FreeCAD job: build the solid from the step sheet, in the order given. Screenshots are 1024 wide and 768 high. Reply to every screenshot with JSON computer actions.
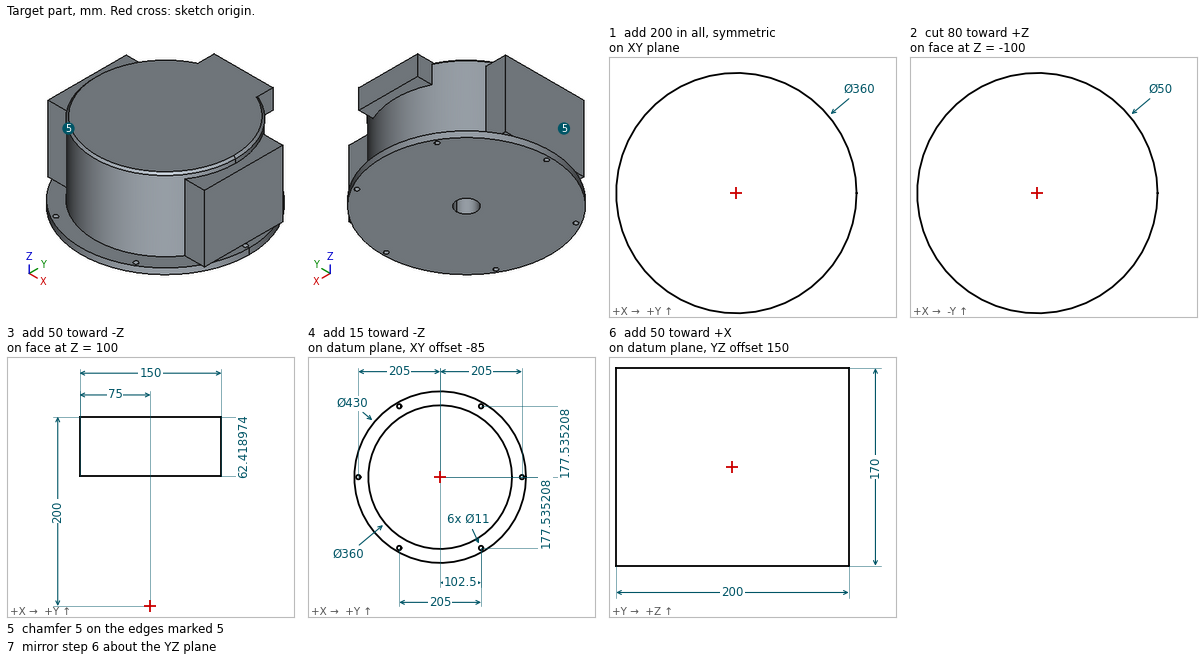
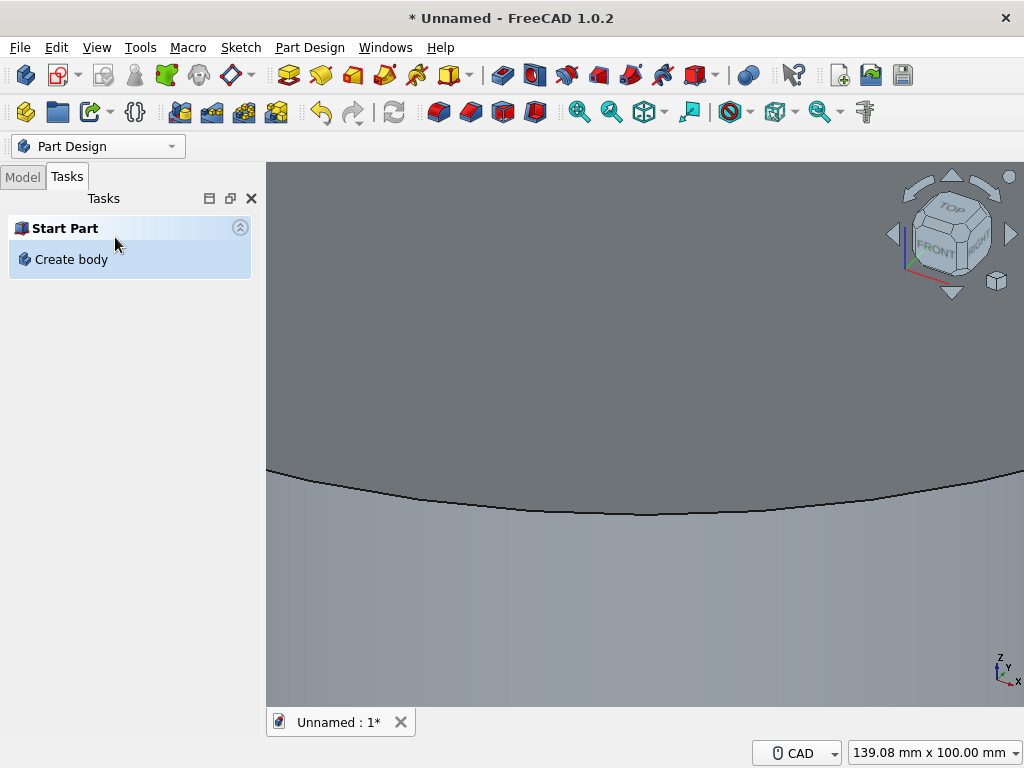
{"action": "left_click", "coordinate": [580, 112]}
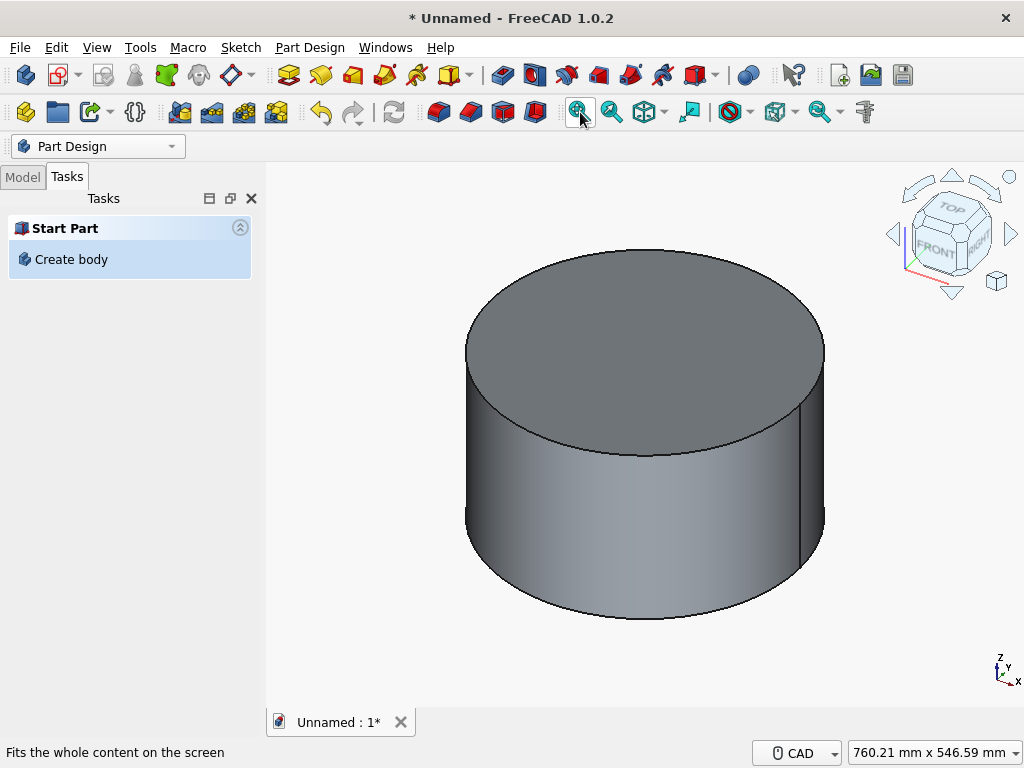
{"action": "key", "text": "5"}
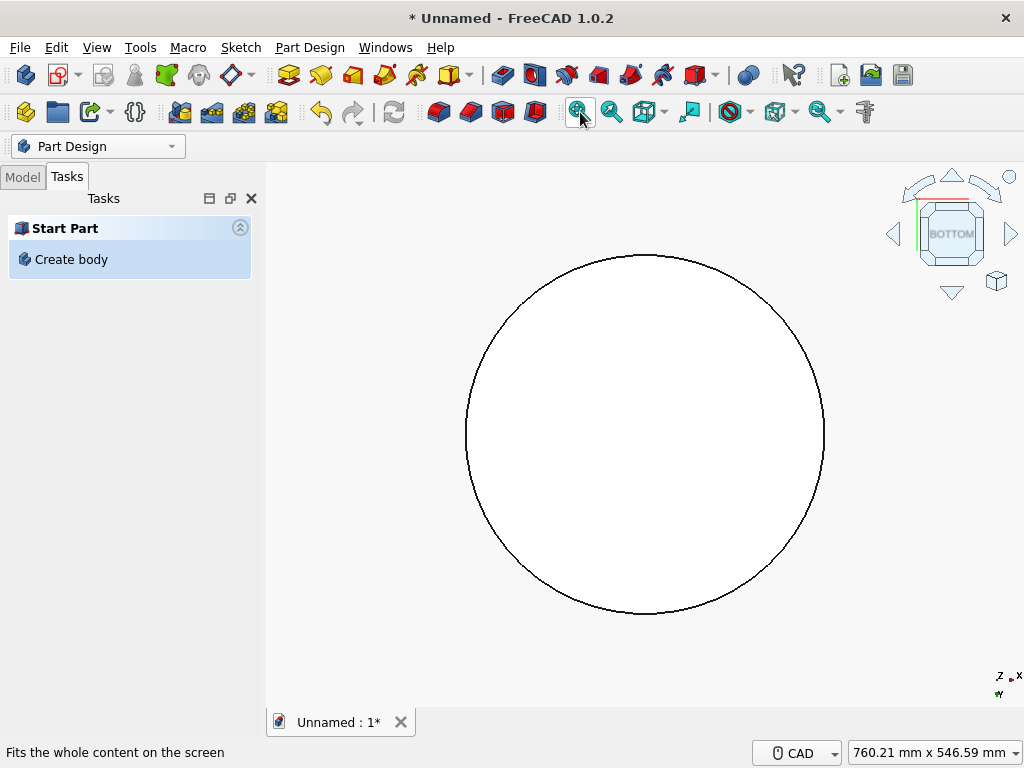
{"action": "left_click", "coordinate": [645, 433]}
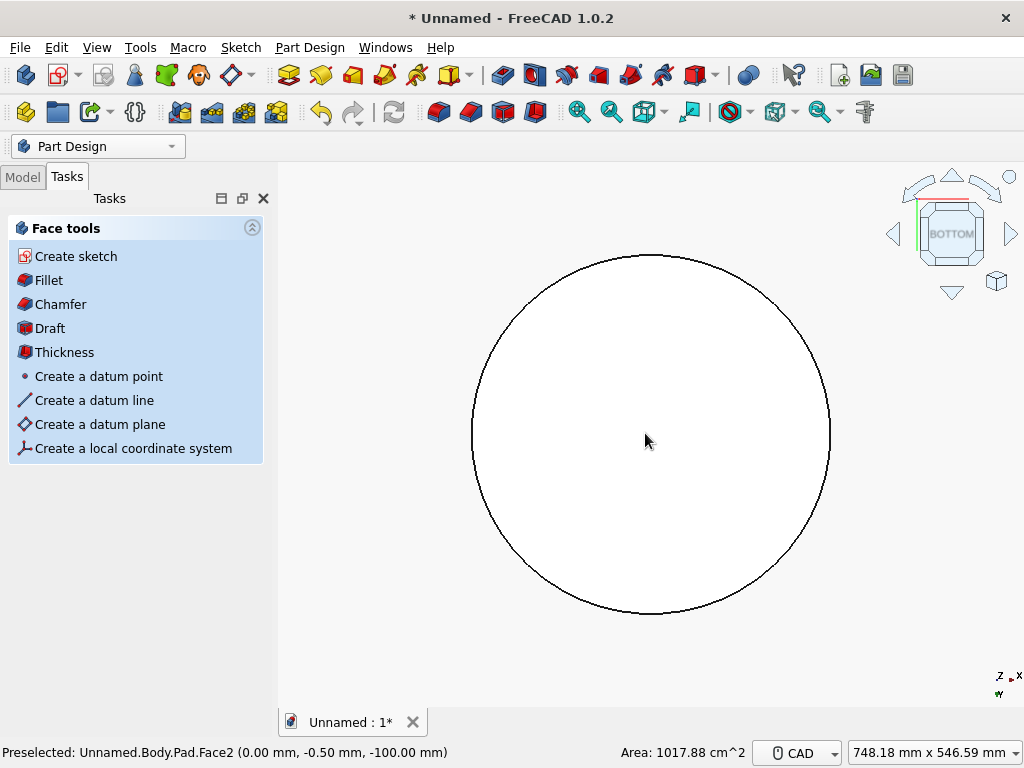
{"action": "left_click", "coordinate": [58, 76]}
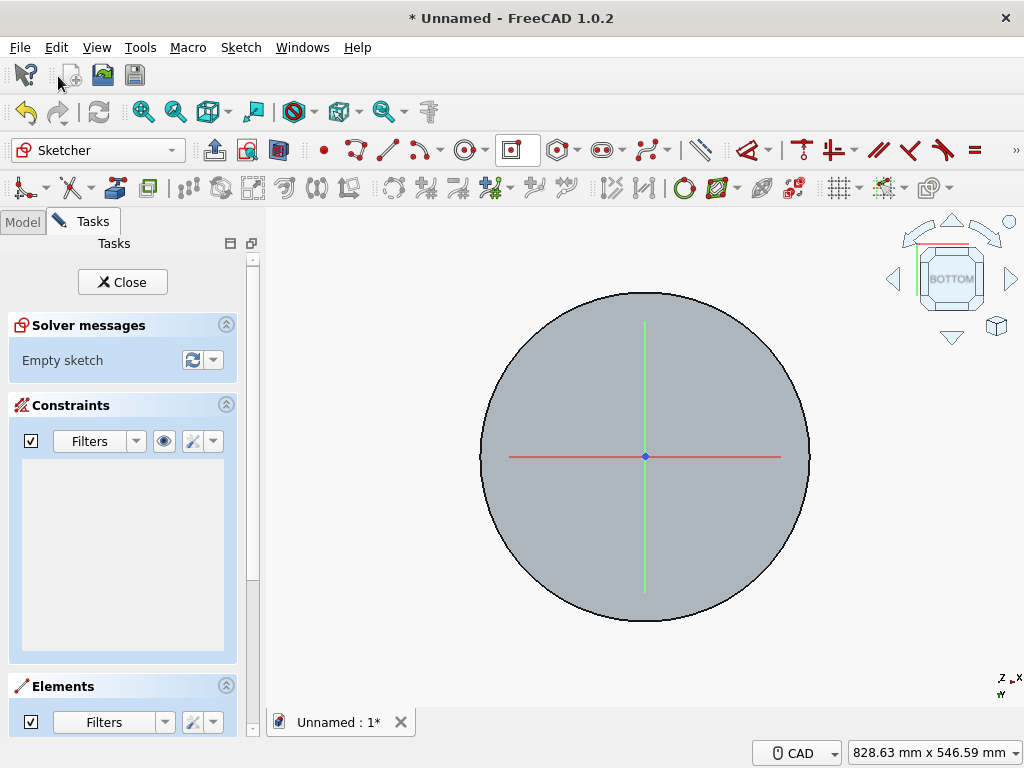
{"action": "scroll", "coordinate": [656, 457], "scroll_direction": "up", "scroll_amount": 10}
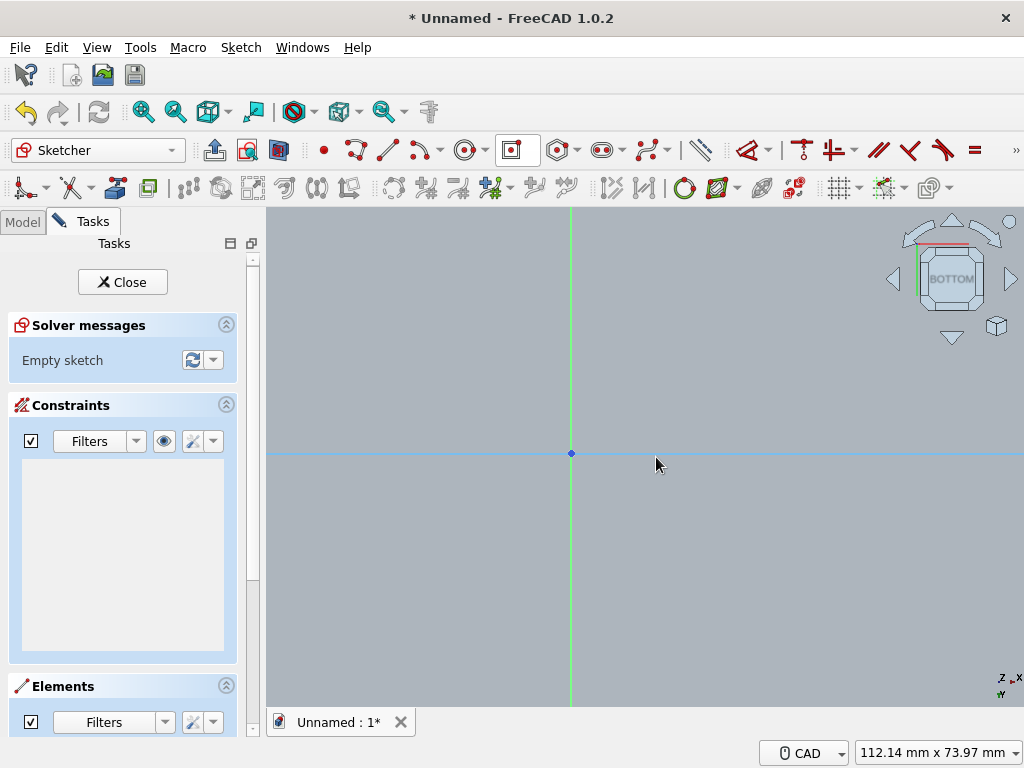
{"action": "key", "text": "g c"}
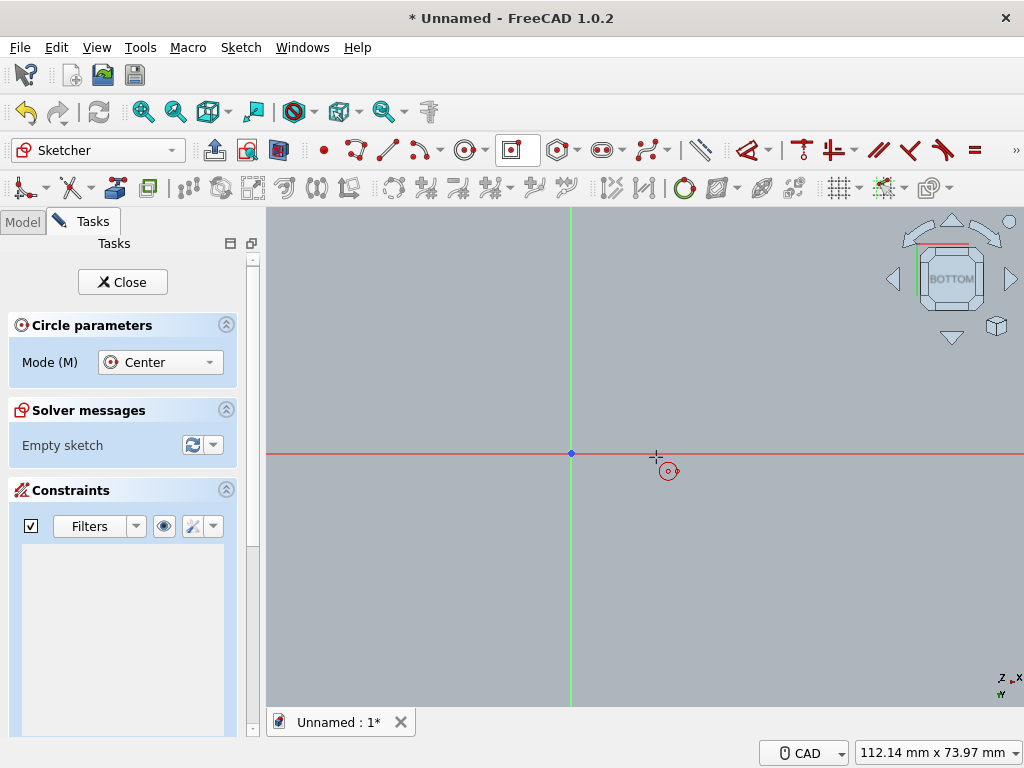
{"action": "left_click", "coordinate": [571, 454]}
{"action": "mouse_move", "coordinate": [691, 334]}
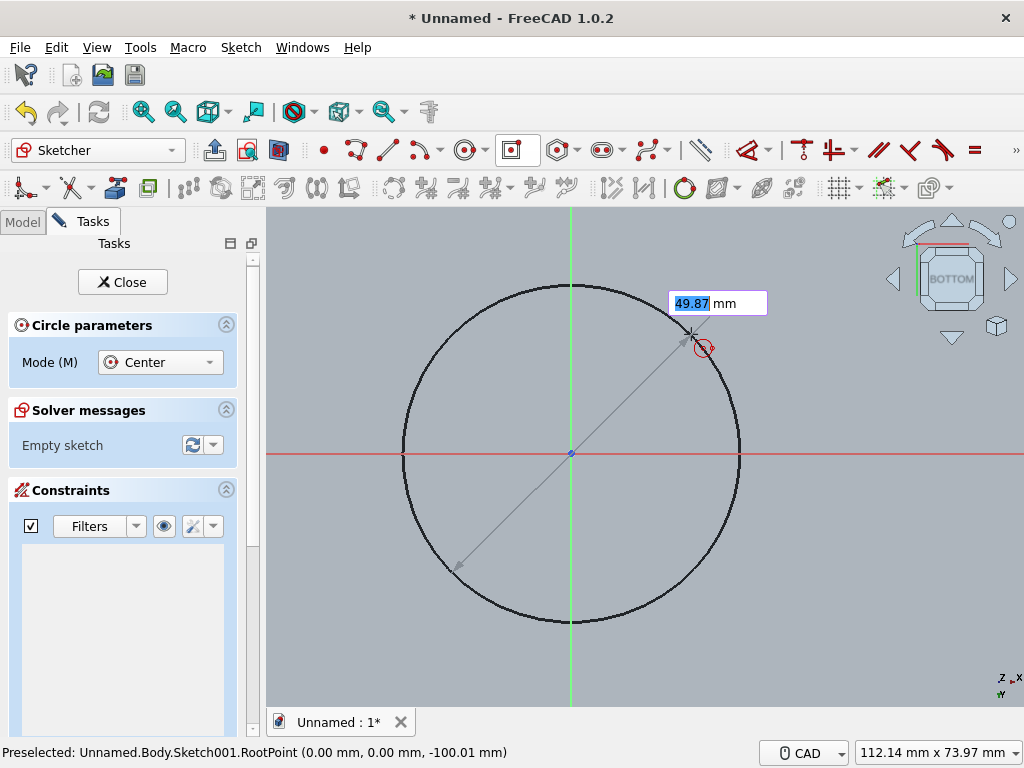
{"action": "type", "text": "50"}
{"action": "key", "text": "Return"}
{"action": "key", "text": "Escape"}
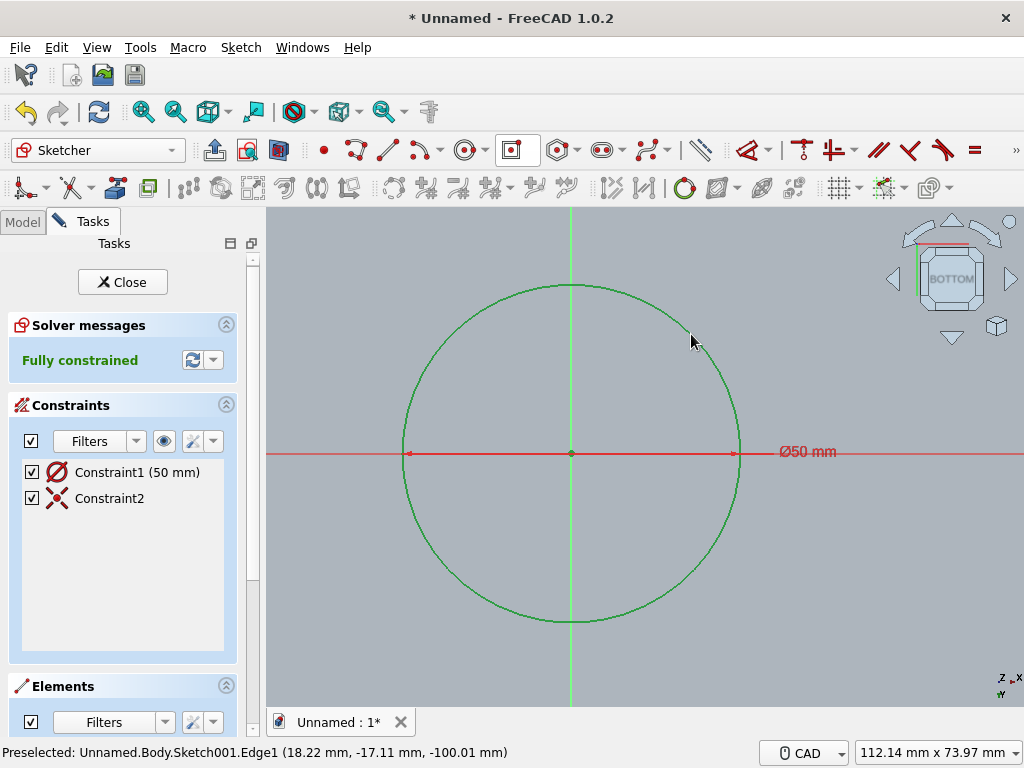
{"action": "left_click", "coordinate": [123, 282]}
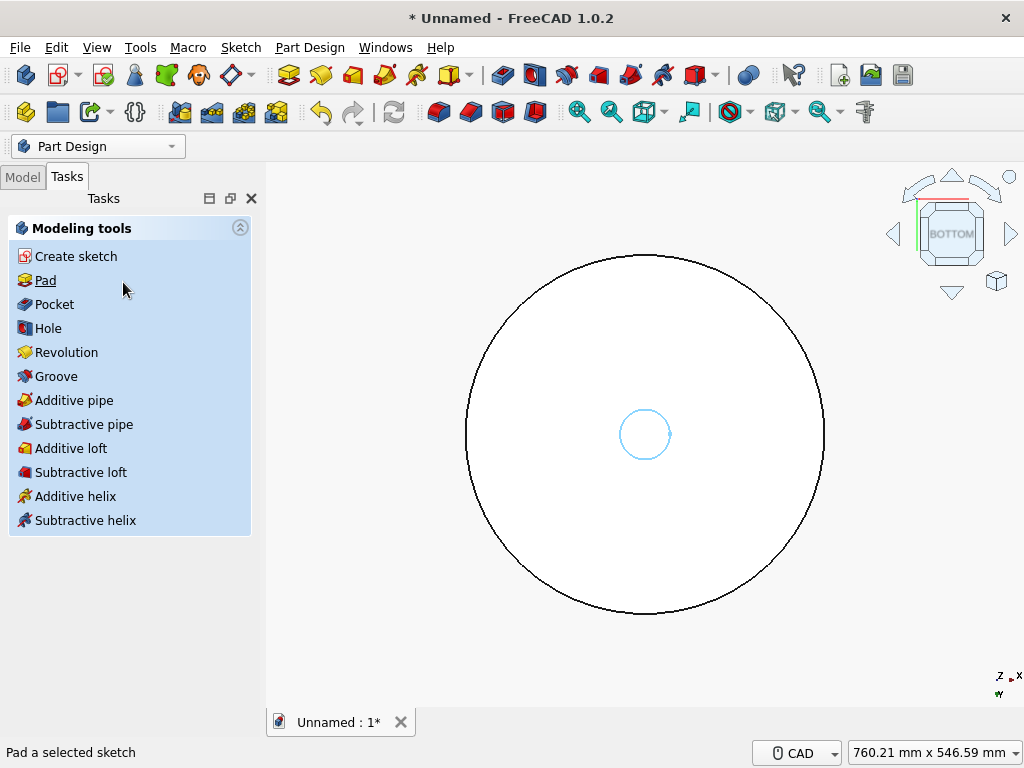
{"action": "left_click", "coordinate": [504, 76]}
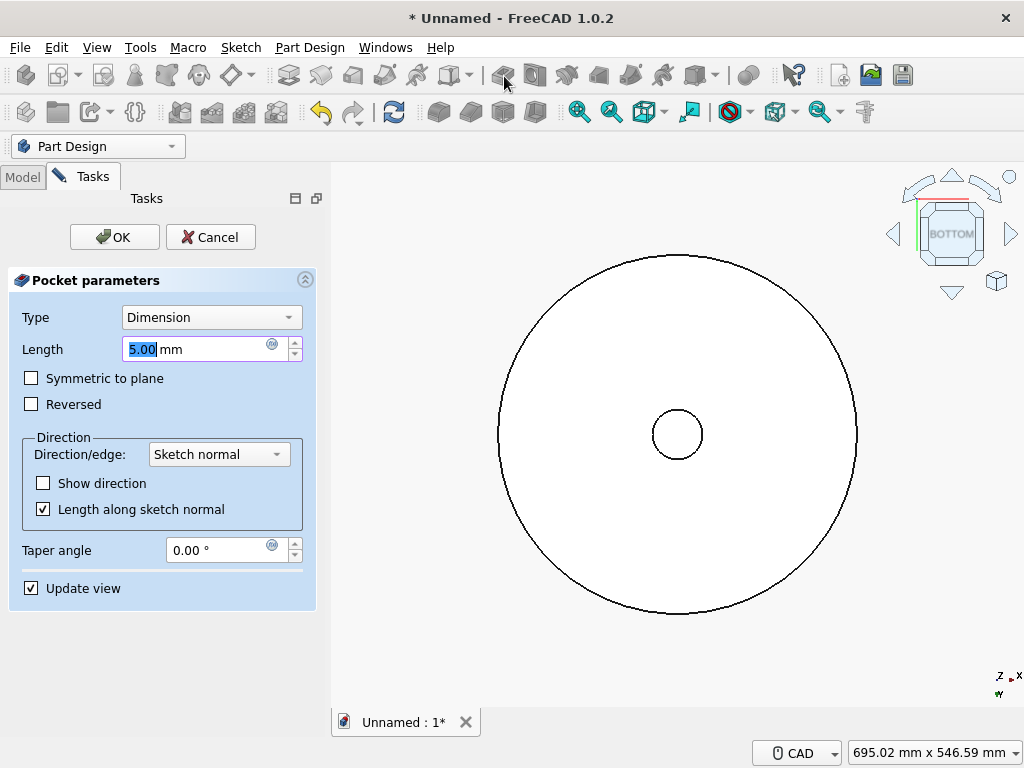
{"action": "type", "text": "80"}
{"action": "key", "text": "Tab"}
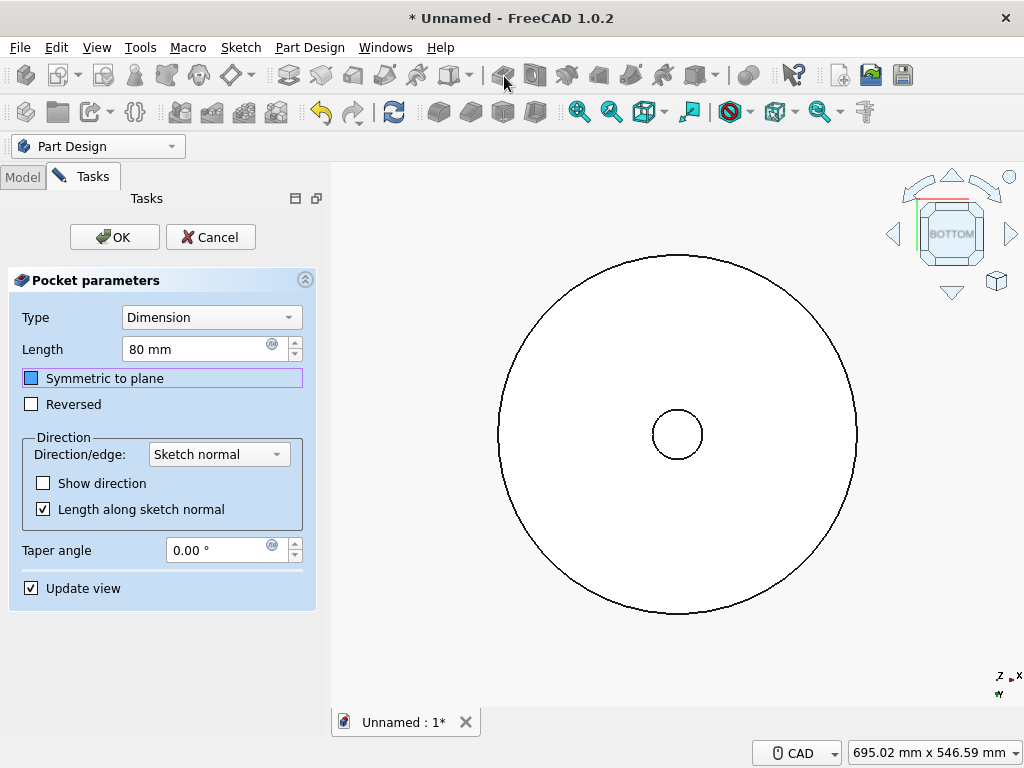
{"action": "left_click", "coordinate": [115, 237]}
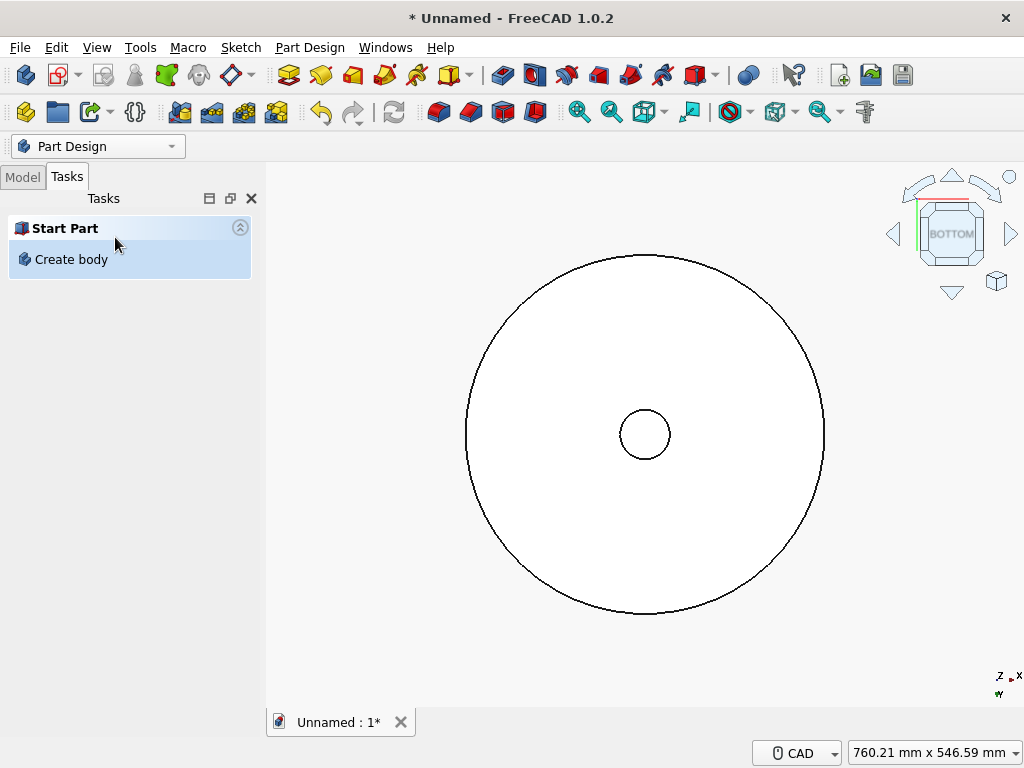
{"action": "key", "text": "0"}